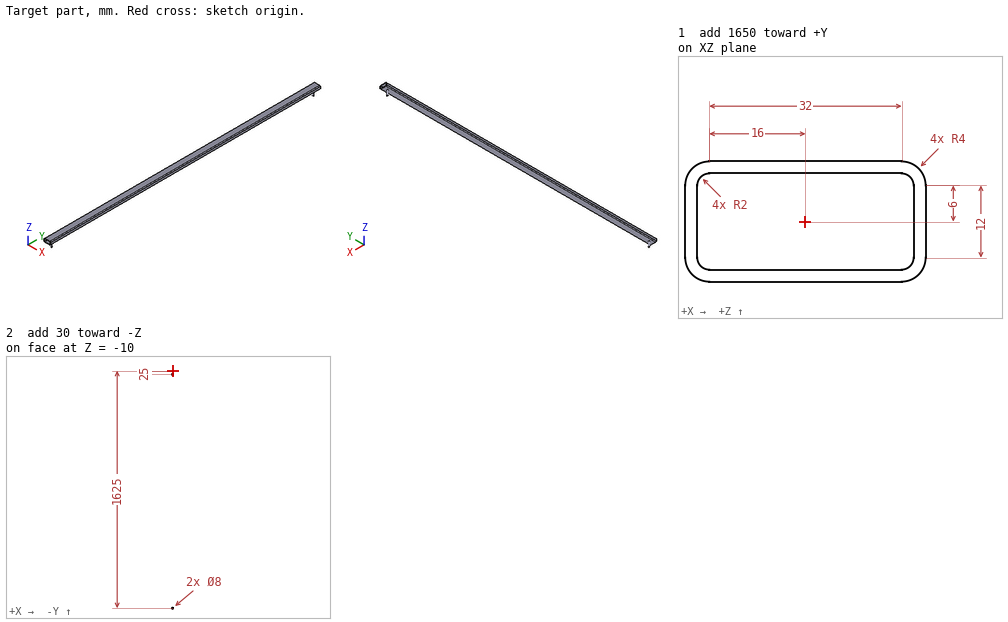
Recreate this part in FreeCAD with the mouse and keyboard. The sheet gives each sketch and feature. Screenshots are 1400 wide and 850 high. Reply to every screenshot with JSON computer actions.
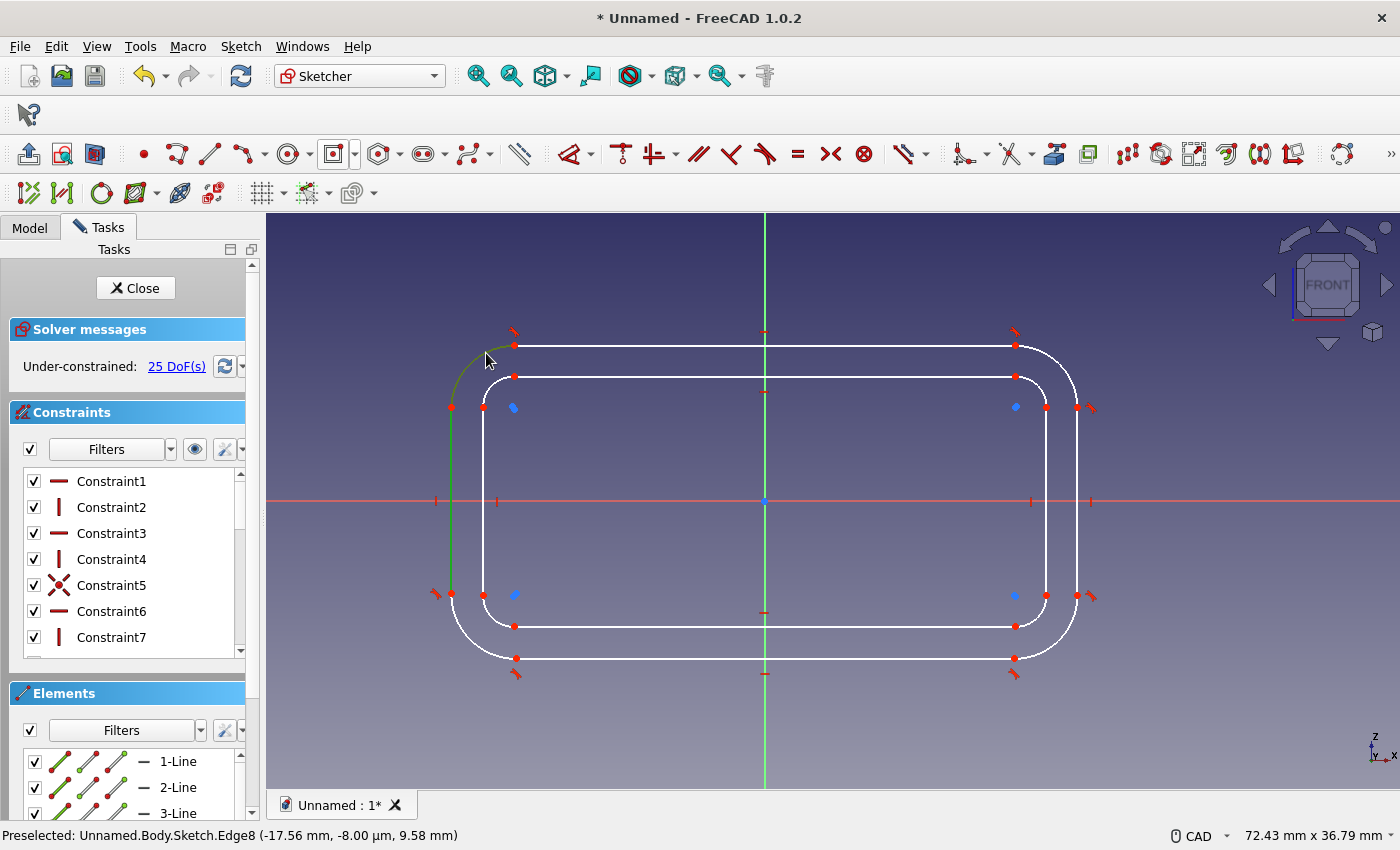
{"action": "left_click", "coordinate": [765, 154]}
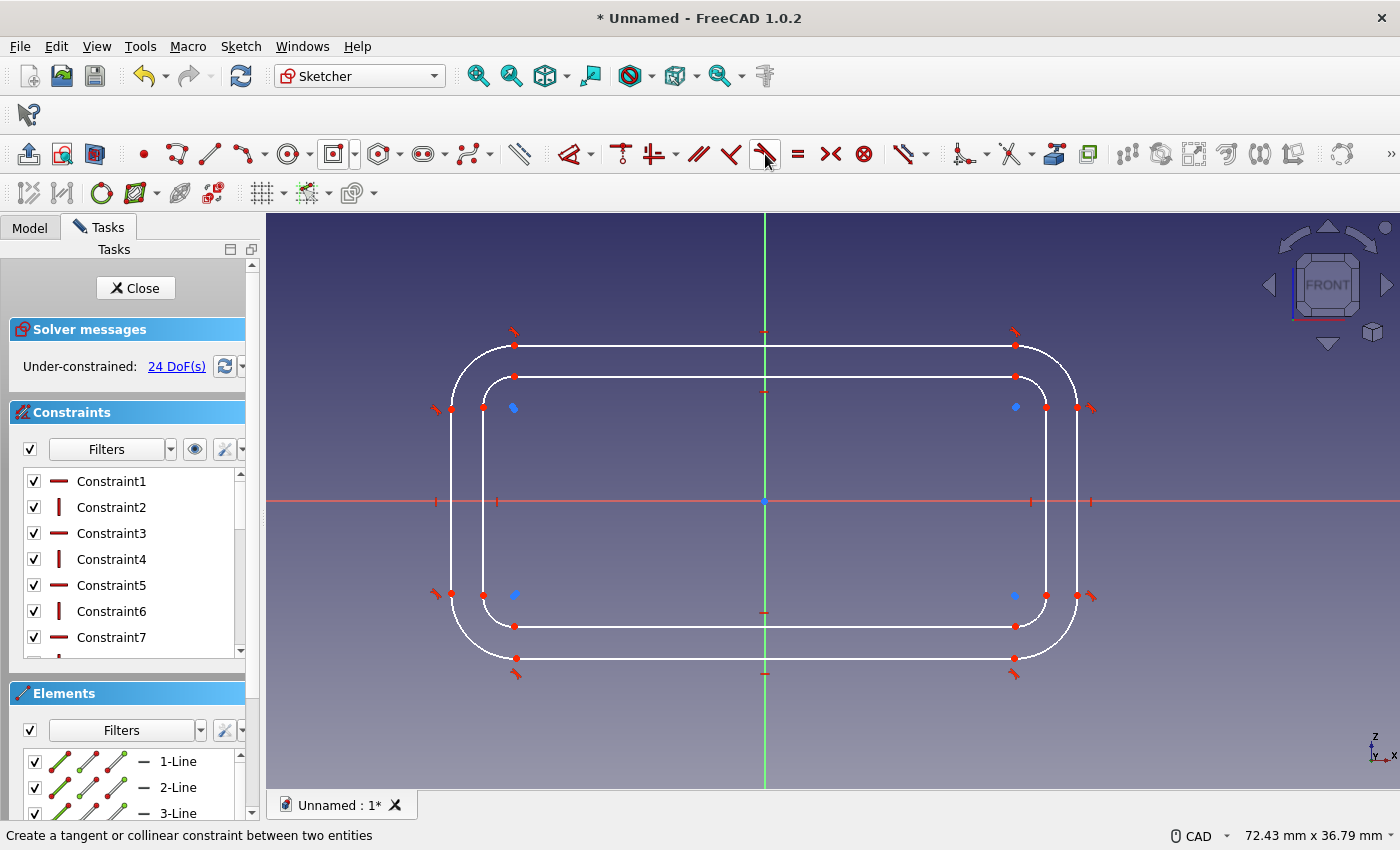
{"action": "left_click", "coordinate": [865, 377]}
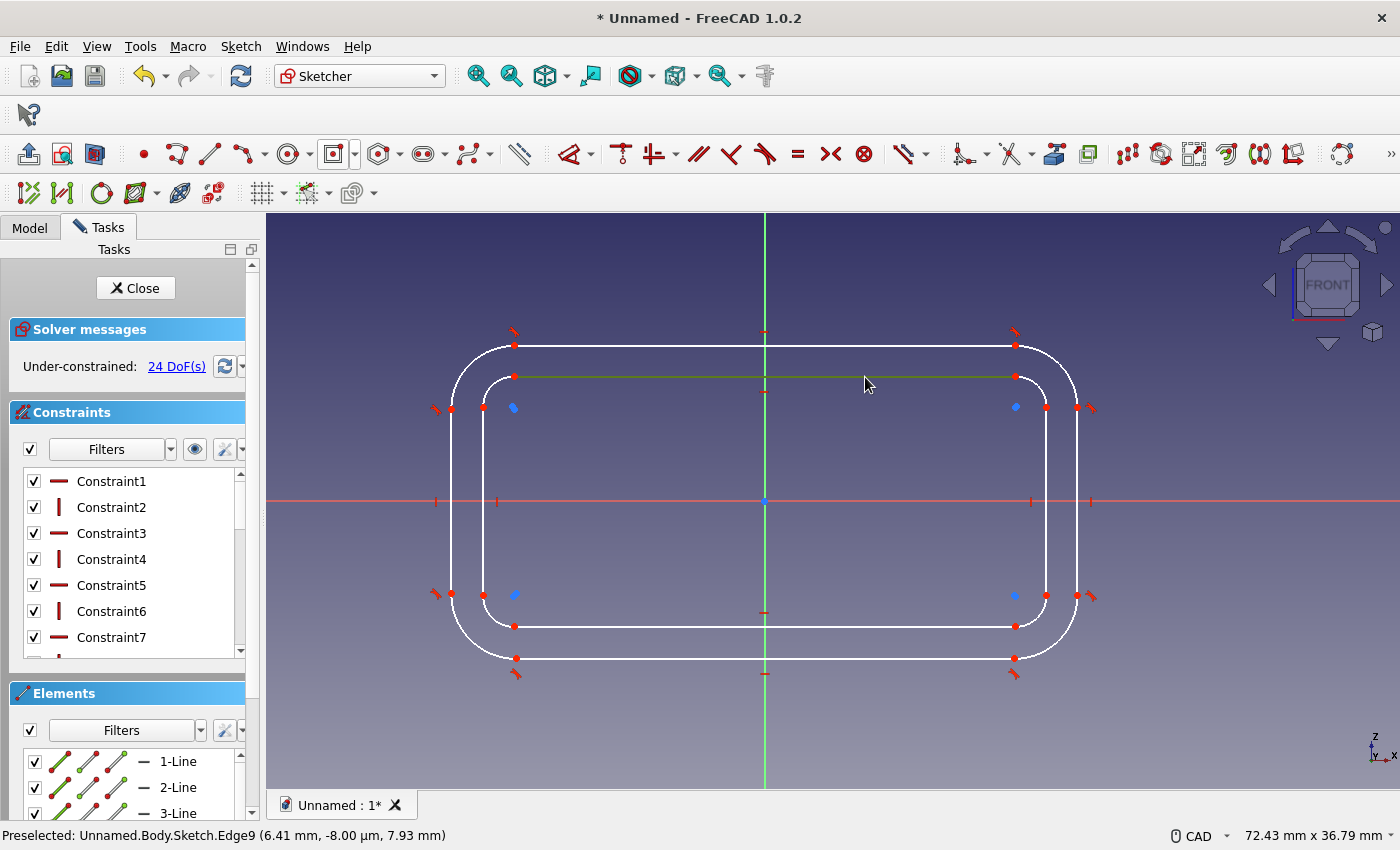
{"action": "left_click", "coordinate": [500, 380]}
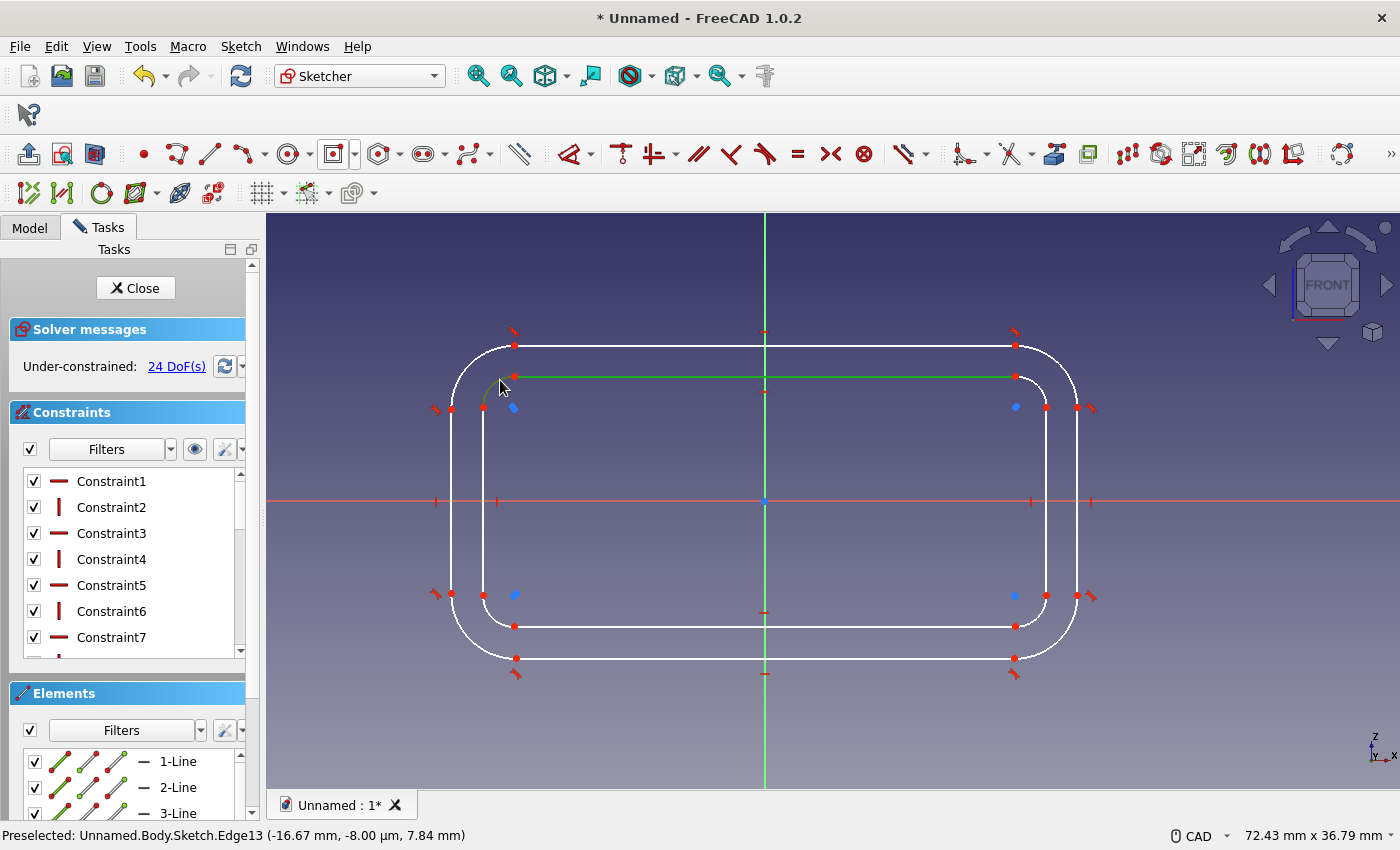
{"action": "left_click", "coordinate": [765, 154]}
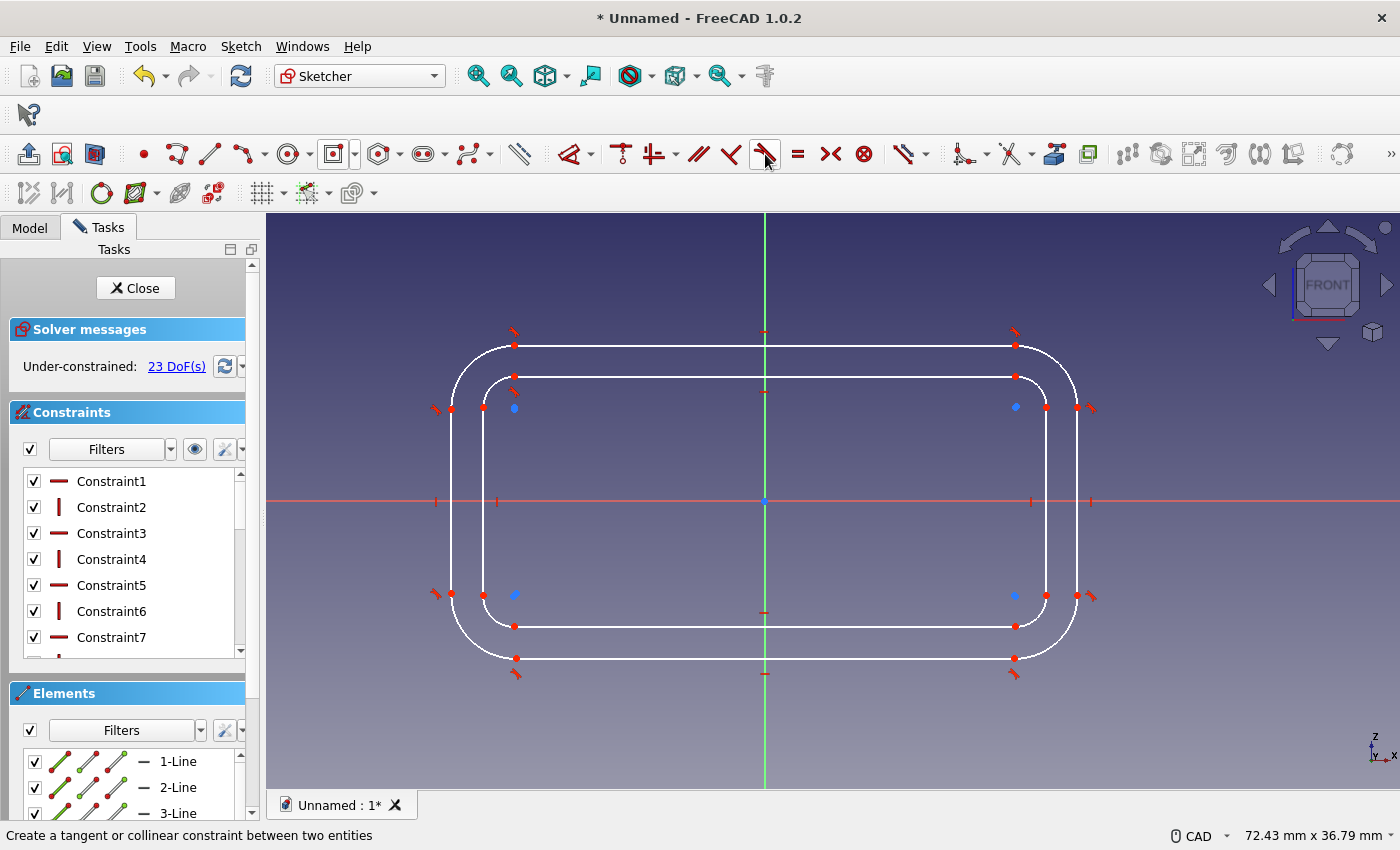
{"action": "left_click", "coordinate": [865, 377]}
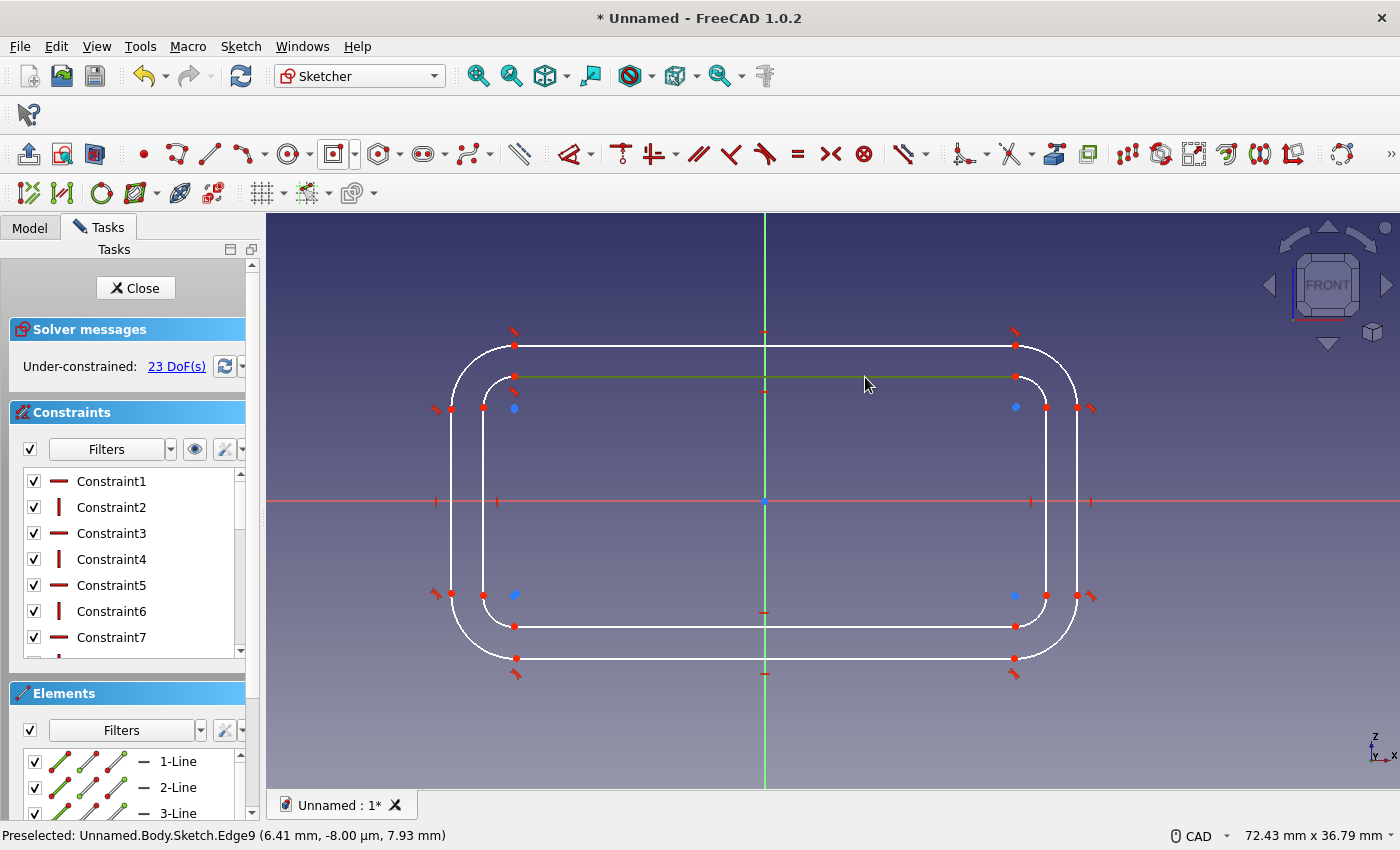
{"action": "left_click", "coordinate": [1043, 394]}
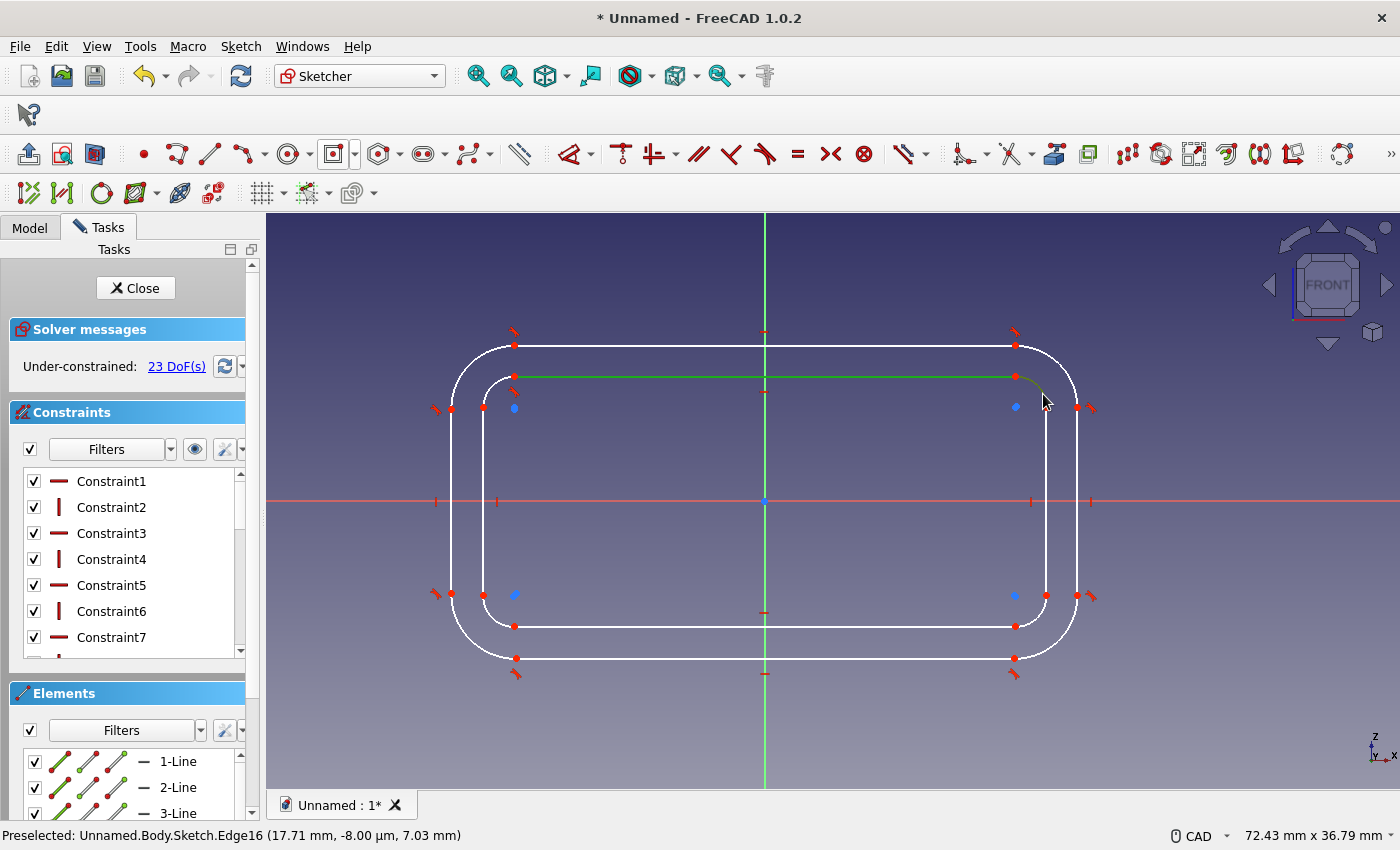
{"action": "left_click", "coordinate": [765, 154]}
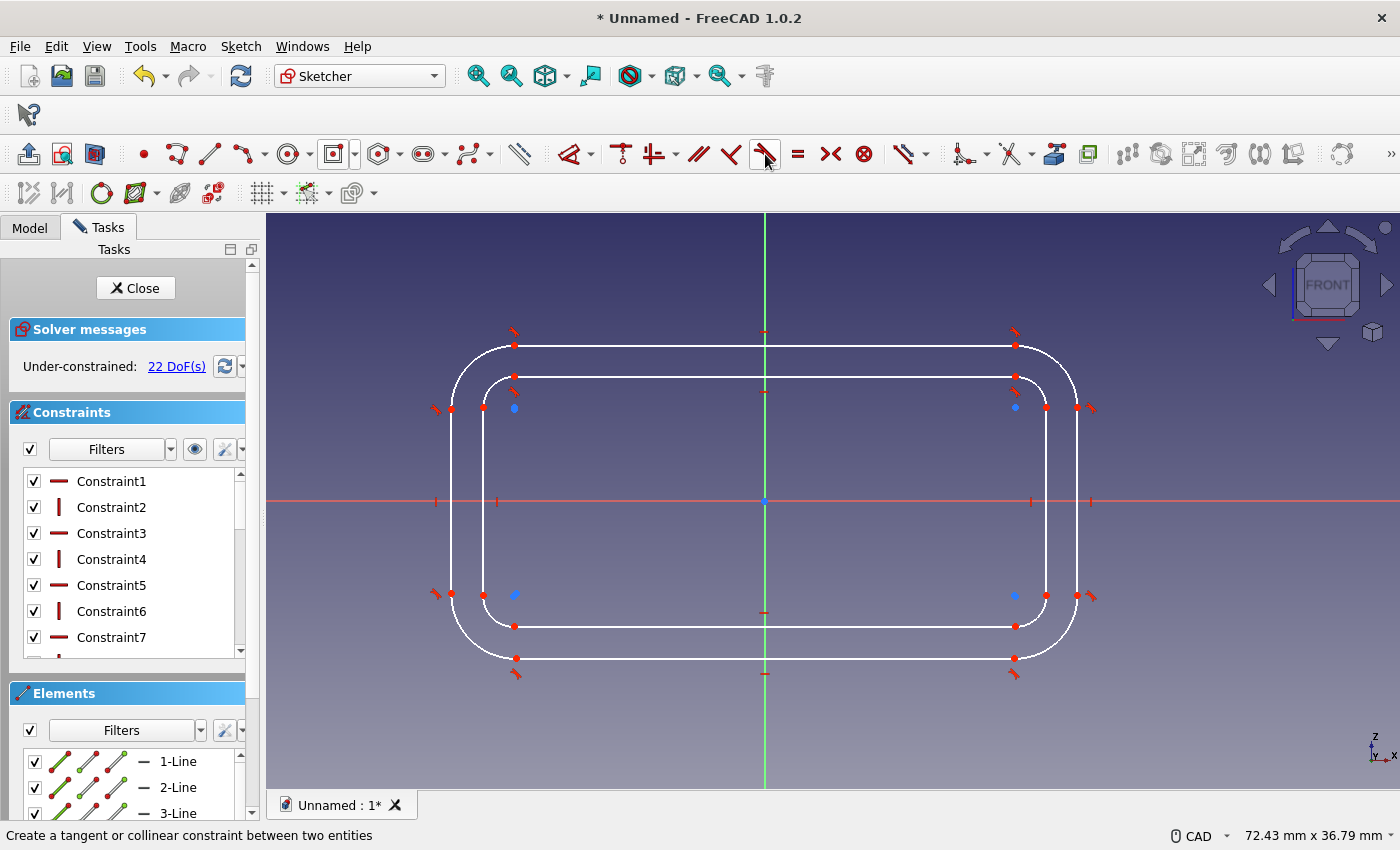
{"action": "left_click", "coordinate": [483, 464]}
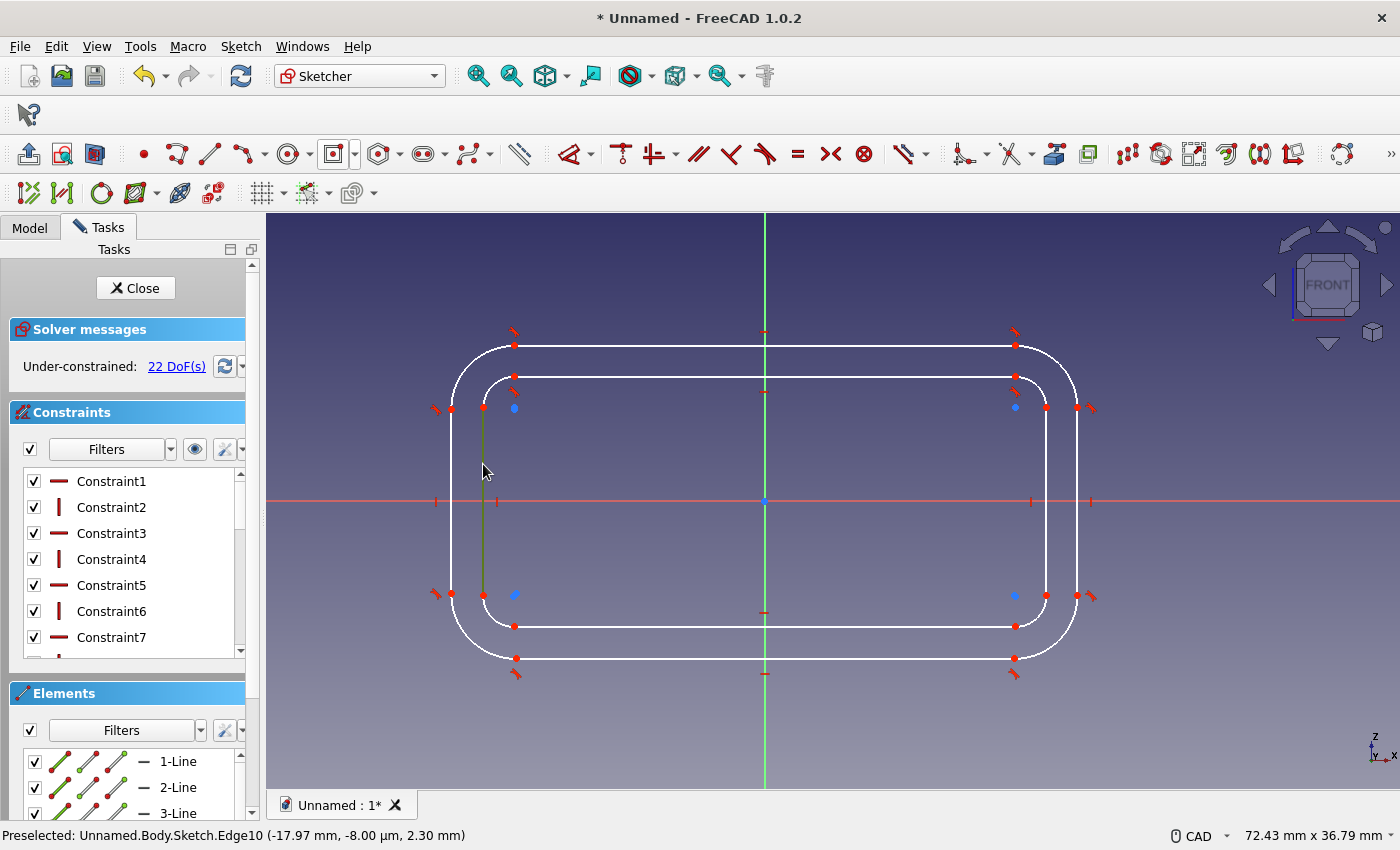
{"action": "left_click", "coordinate": [500, 380]}